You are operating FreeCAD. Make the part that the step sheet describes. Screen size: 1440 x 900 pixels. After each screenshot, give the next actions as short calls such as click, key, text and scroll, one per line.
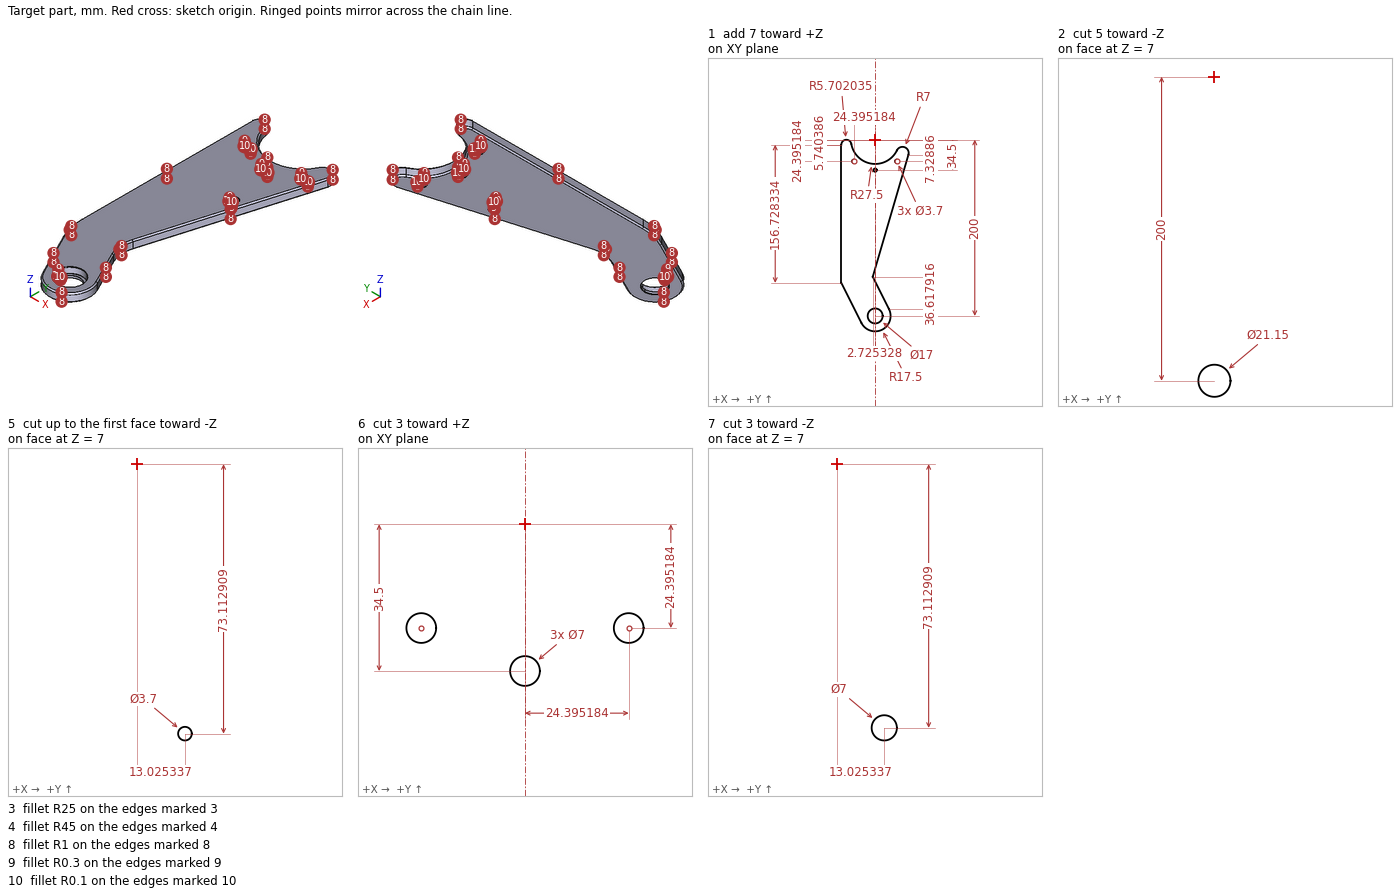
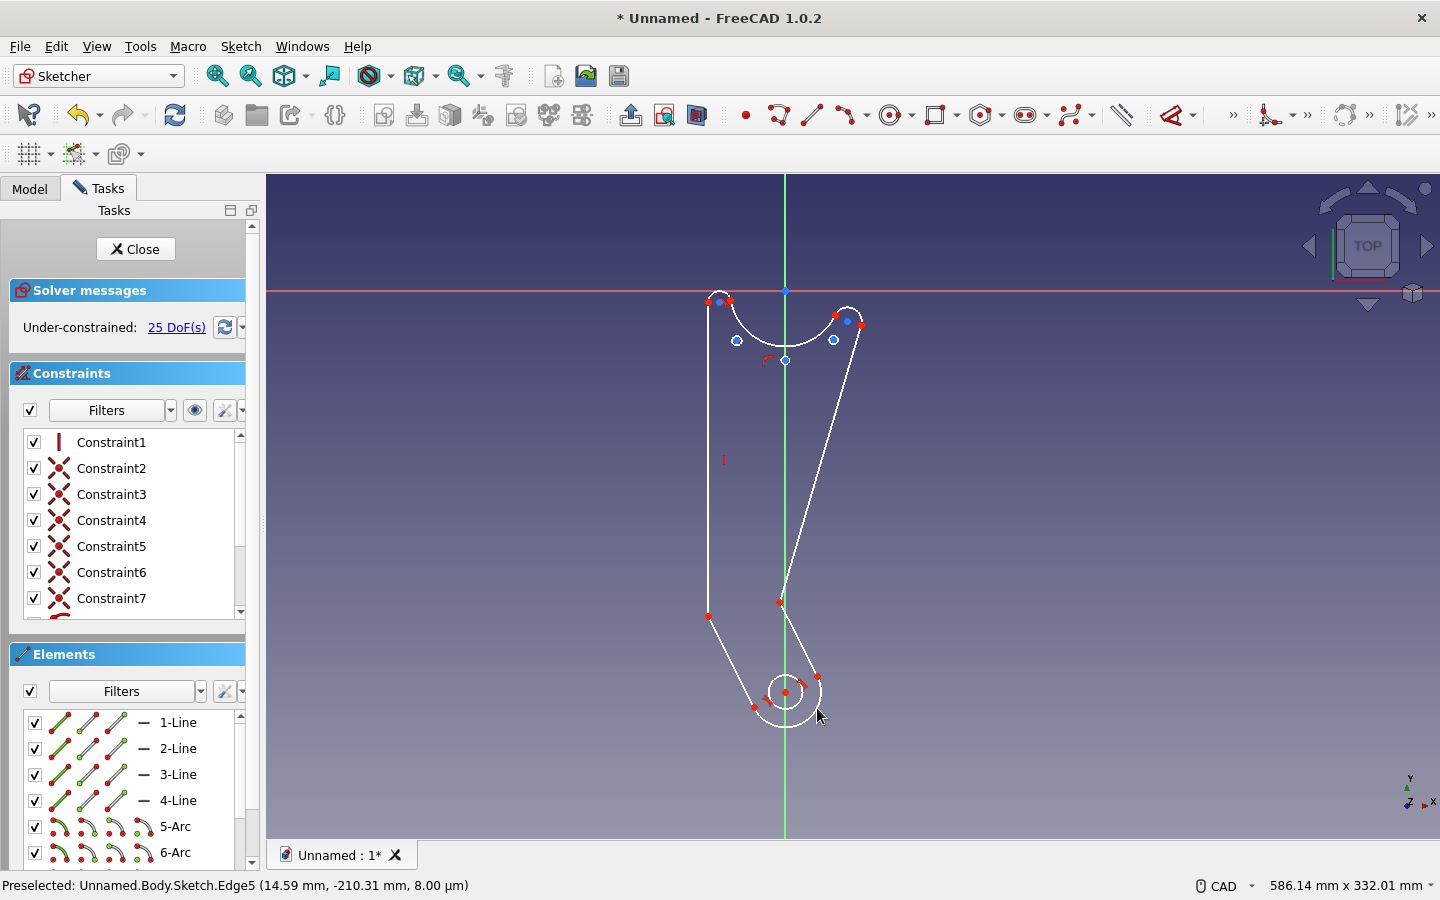
click(804, 519)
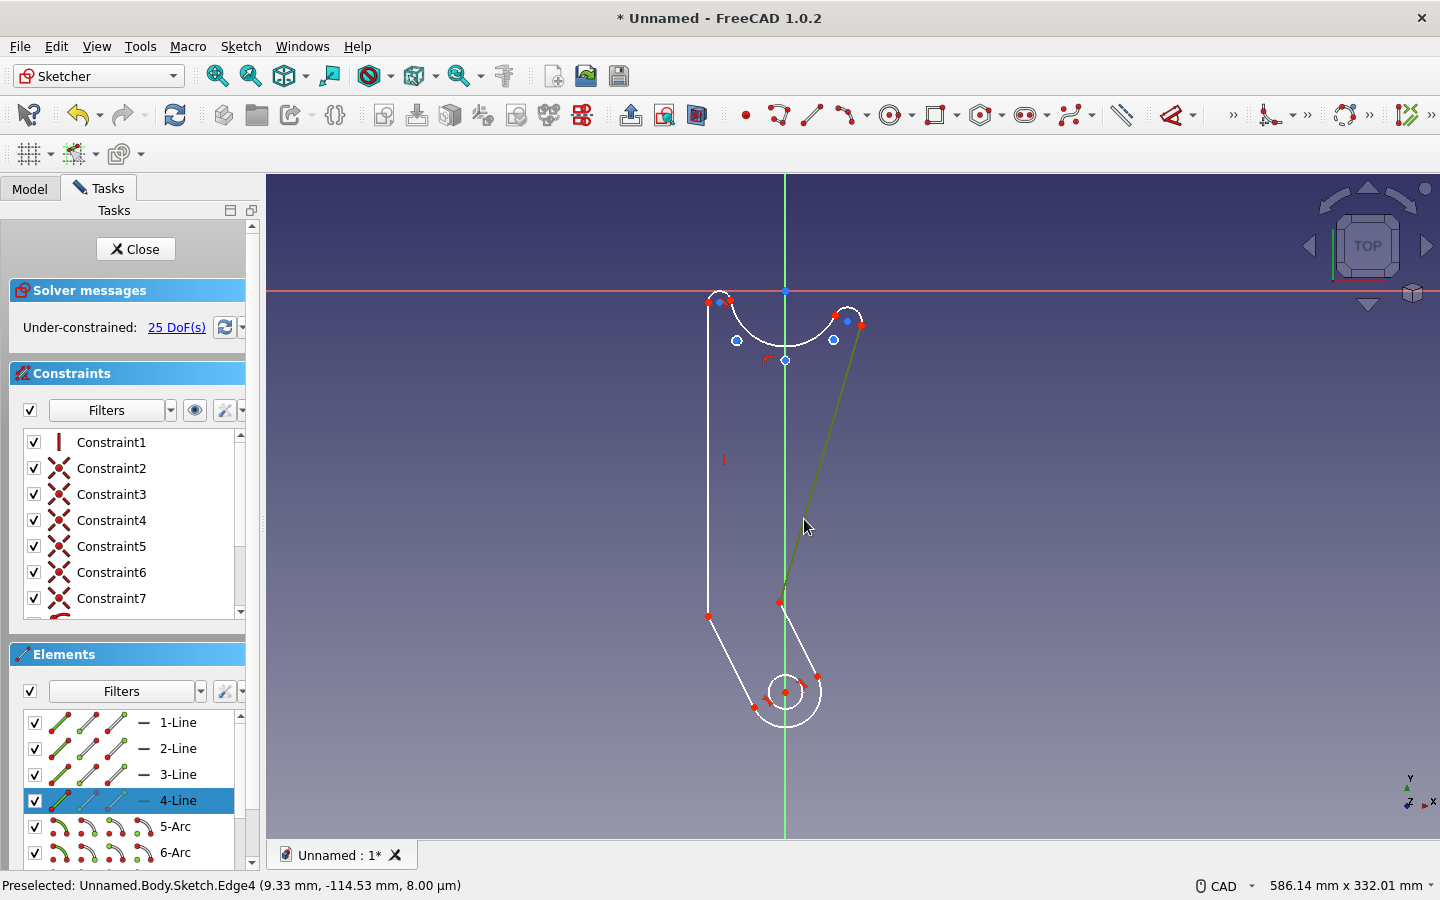
click(859, 313)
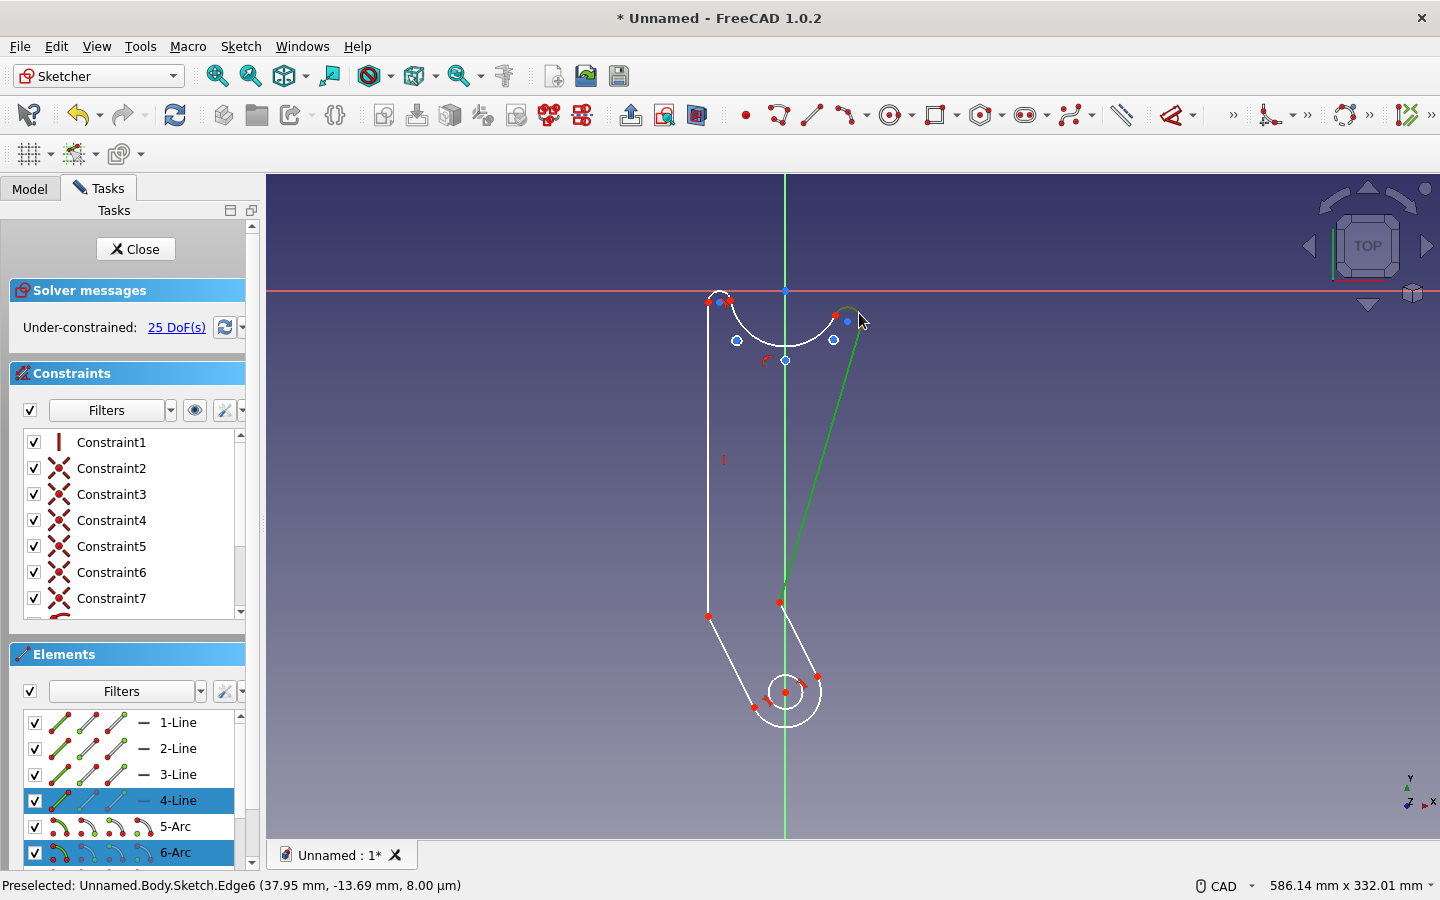
key(t)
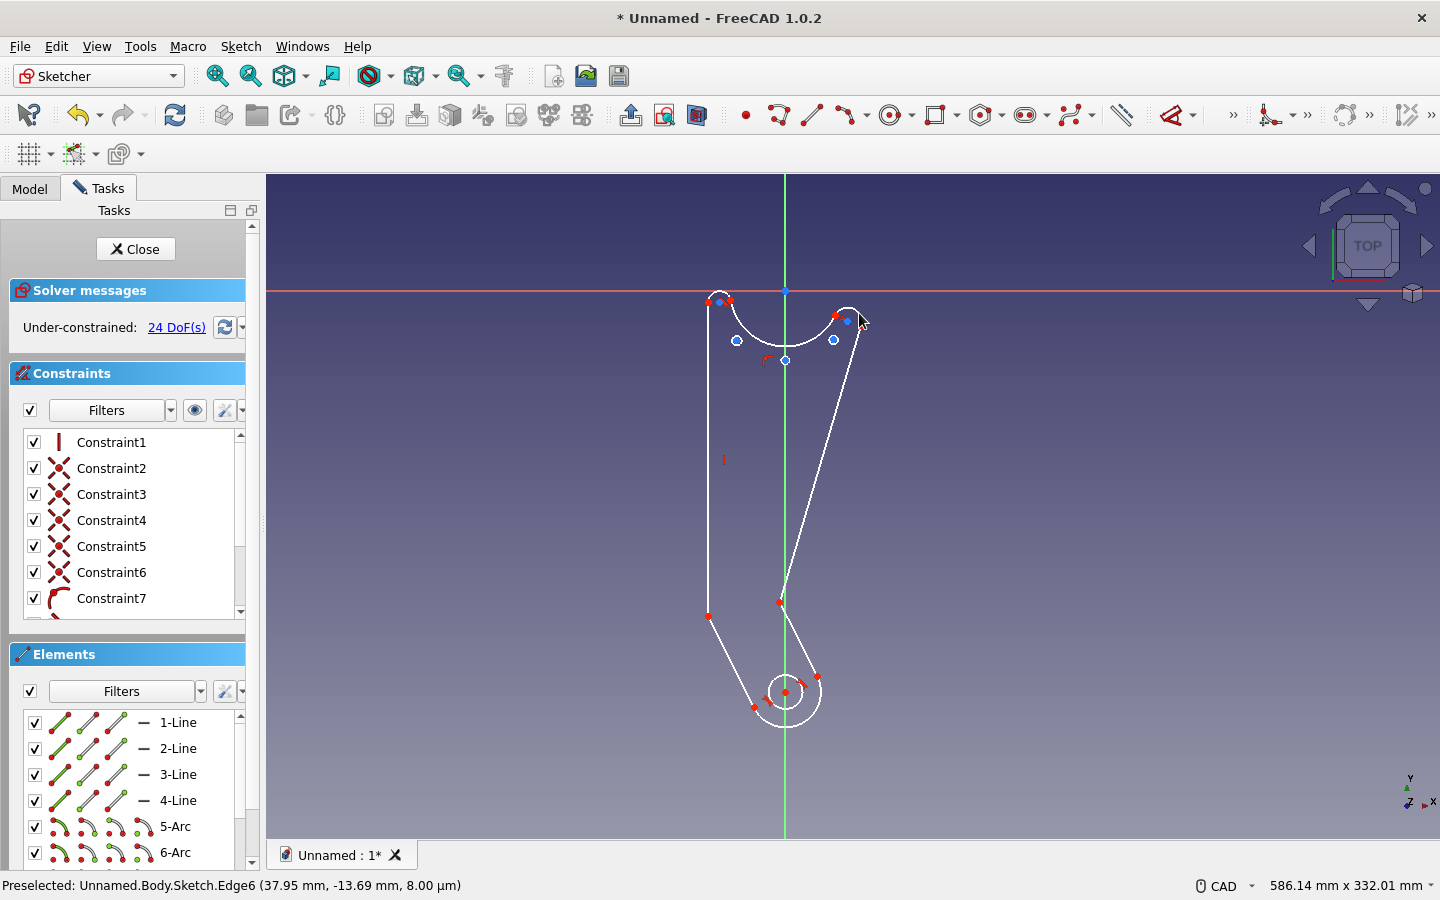
click(859, 314)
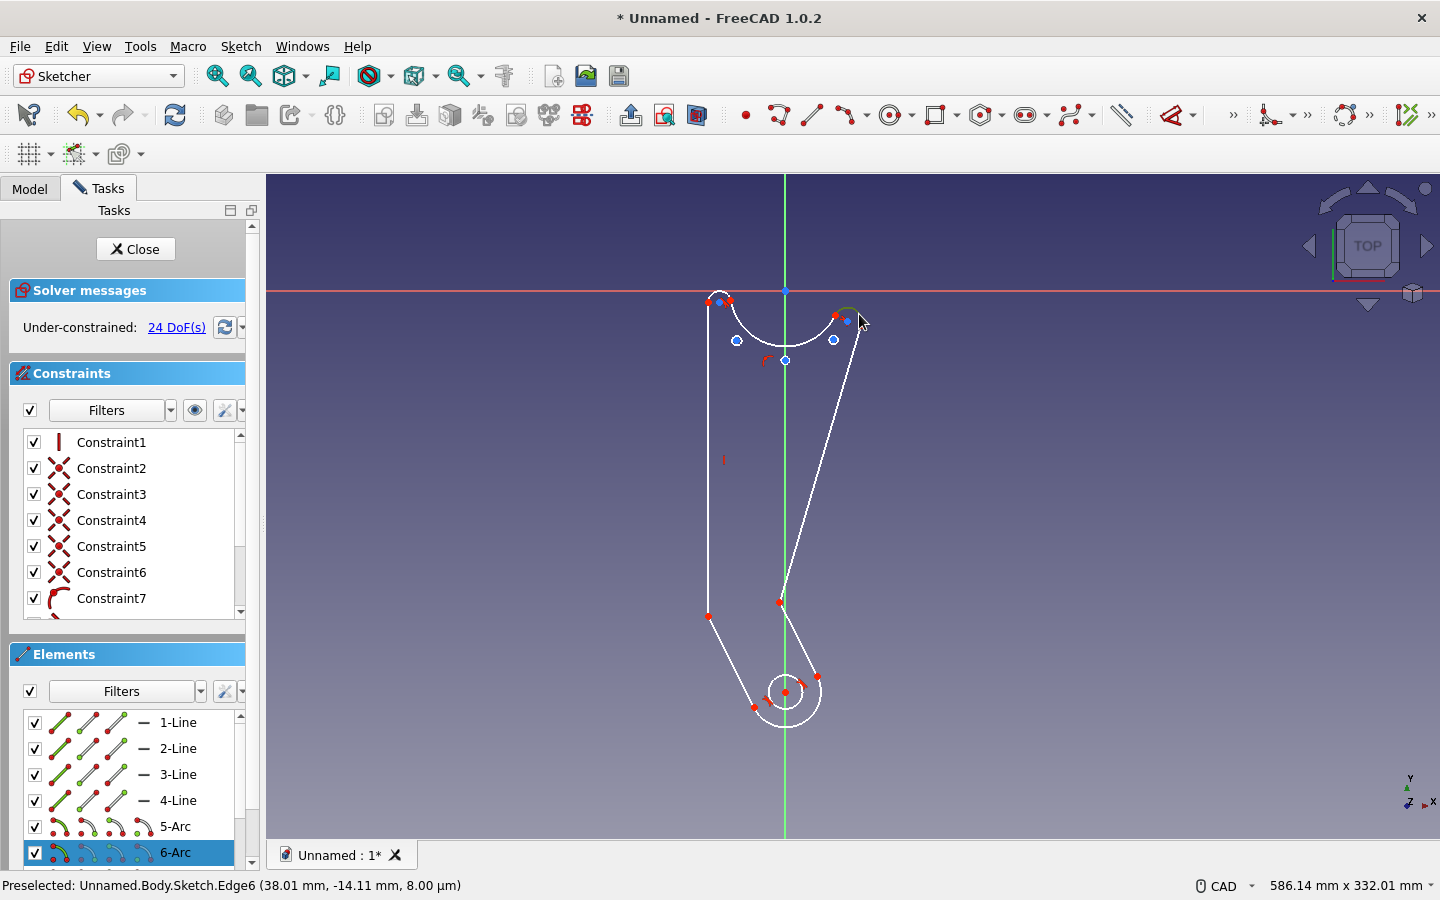
click(752, 335)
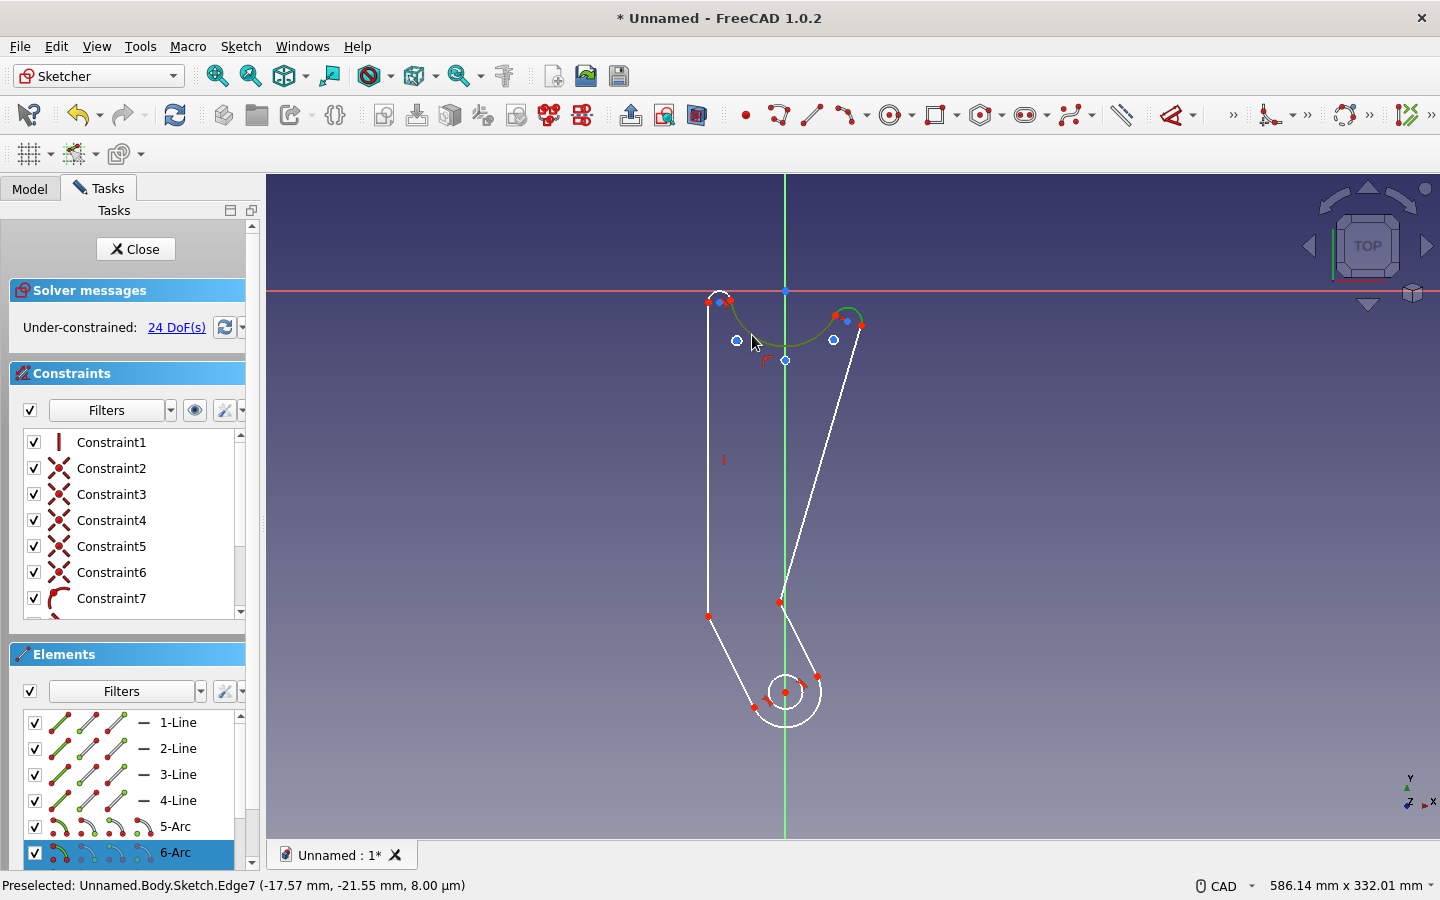
key(t)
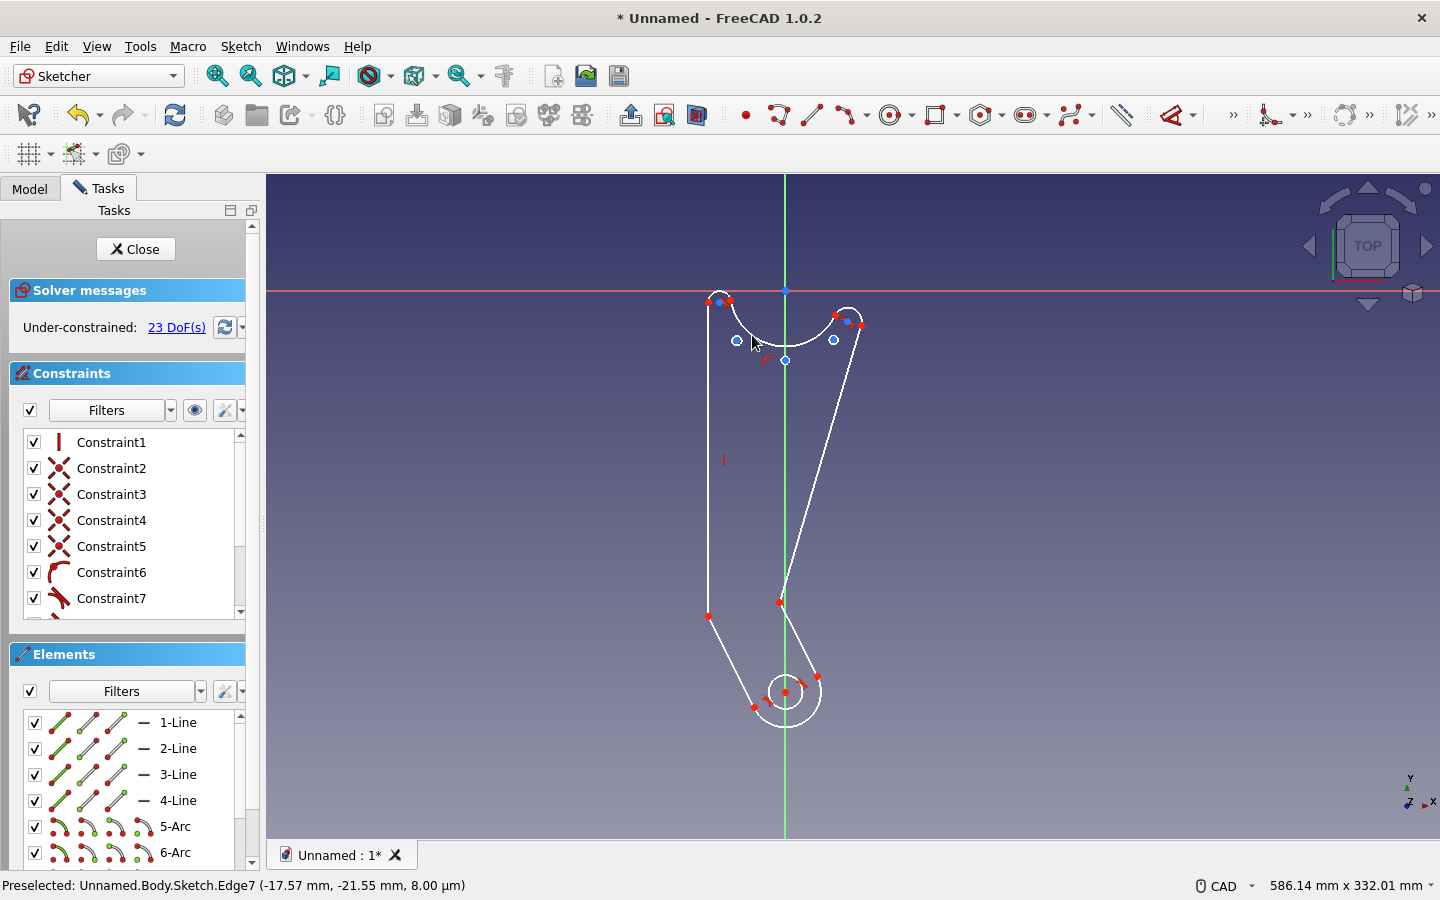
click(752, 335)